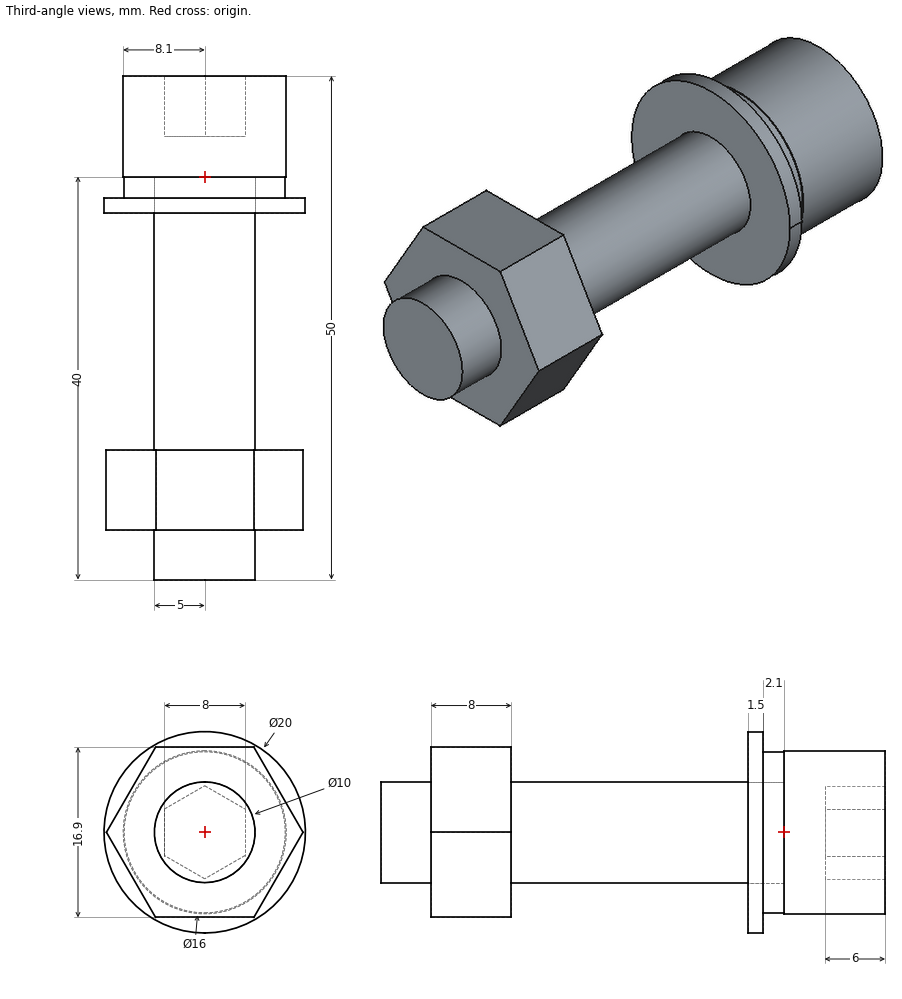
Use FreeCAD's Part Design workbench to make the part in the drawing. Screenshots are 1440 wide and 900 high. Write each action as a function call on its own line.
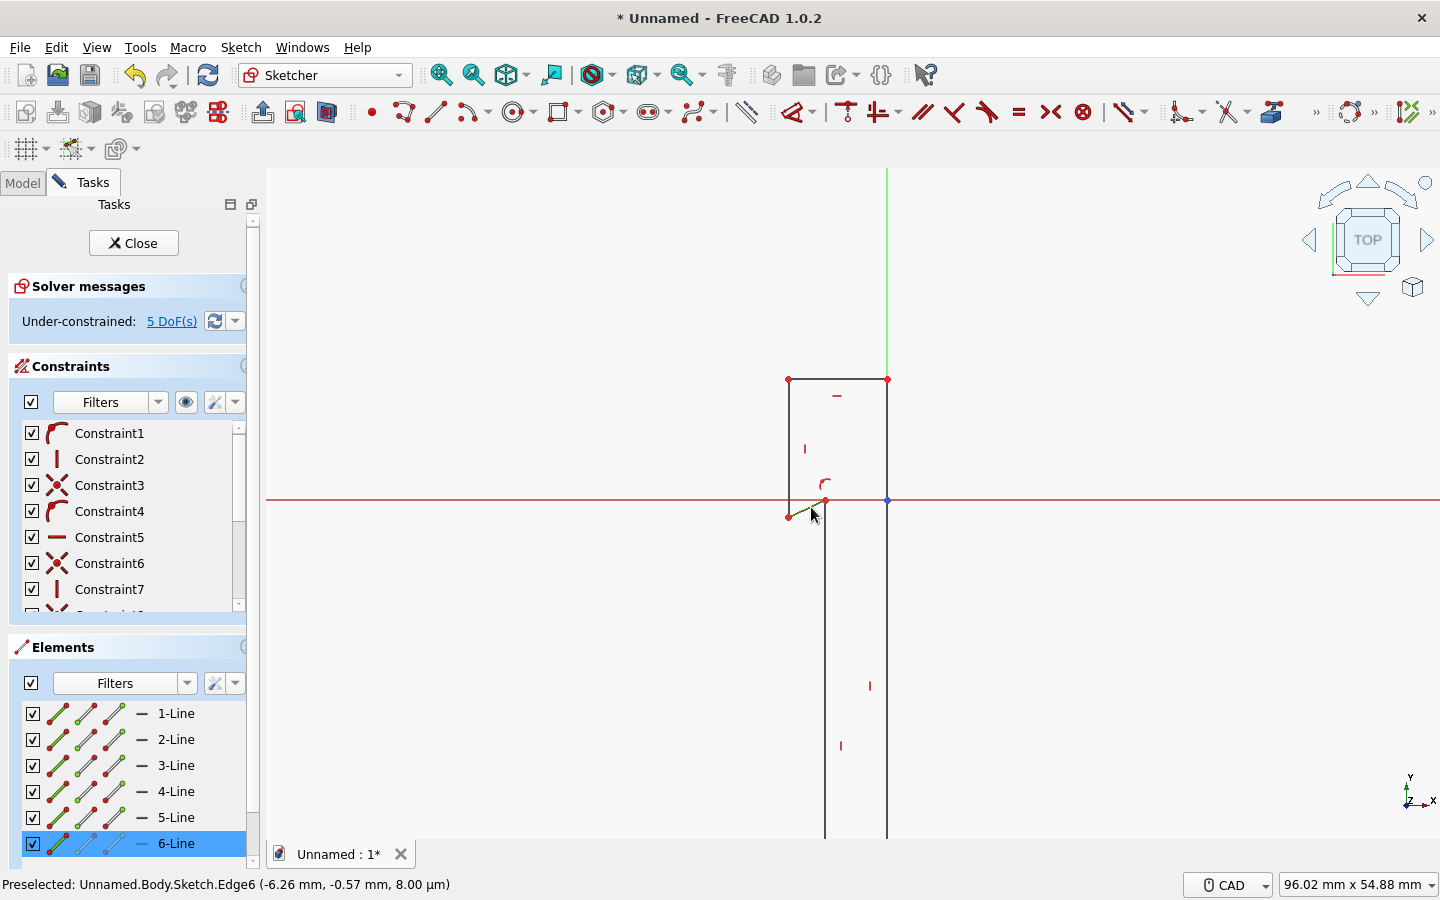
click(900, 112)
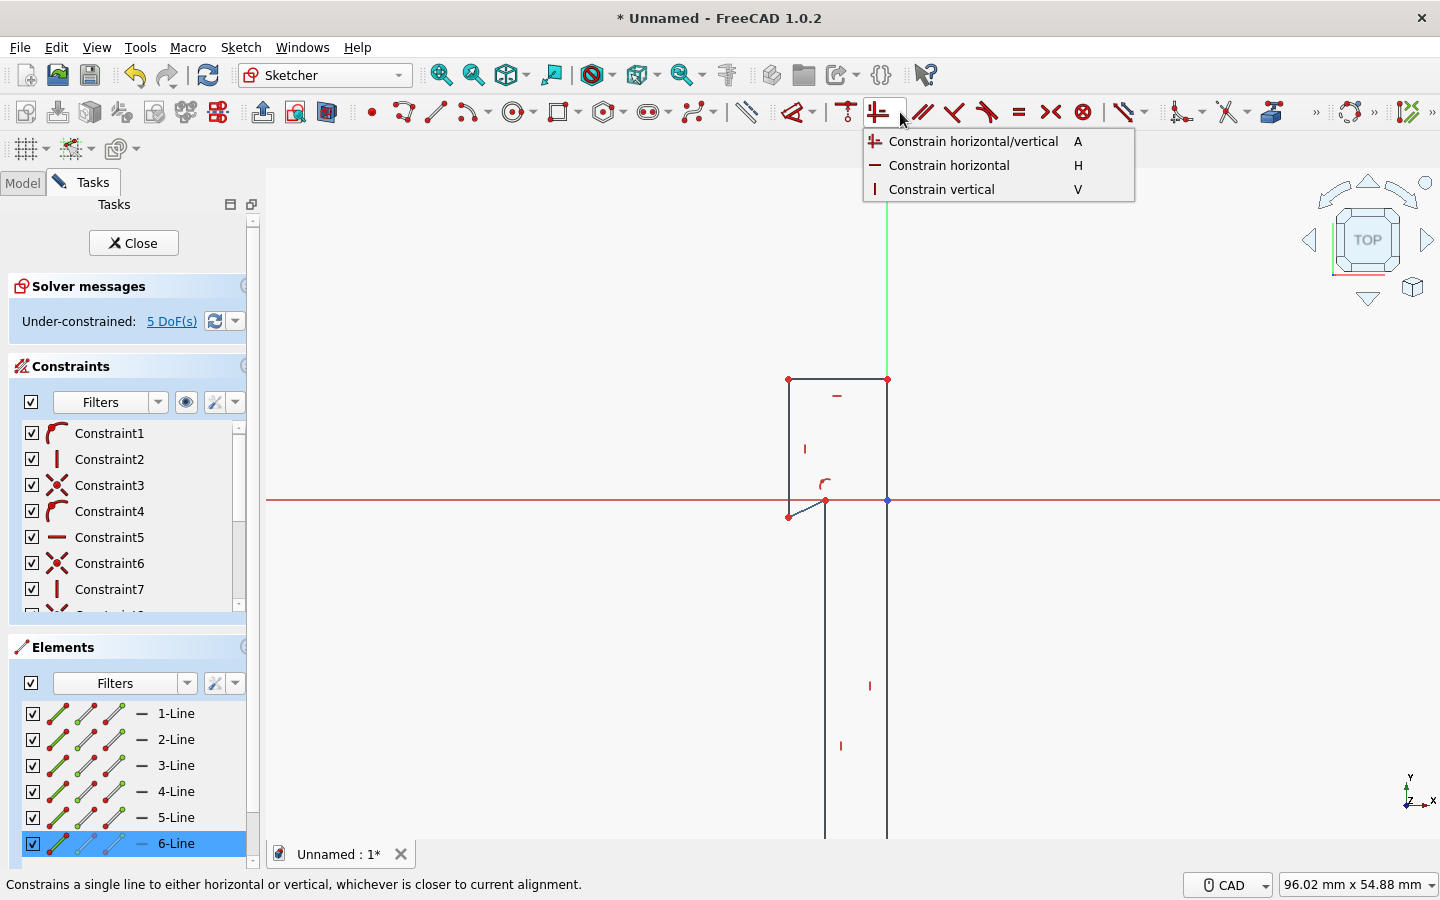
click(999, 165)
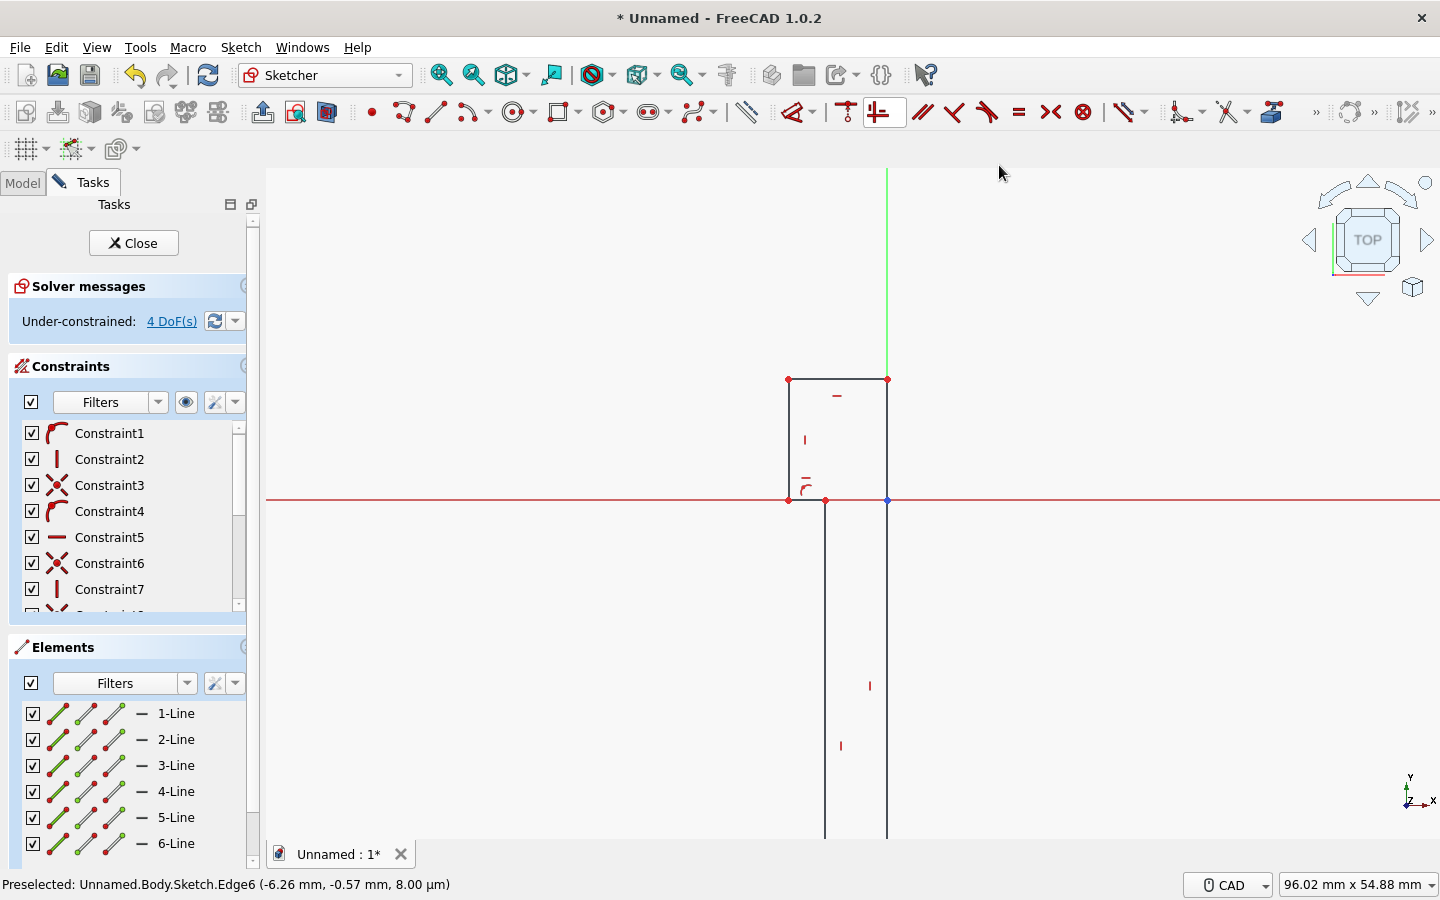
click(792, 112)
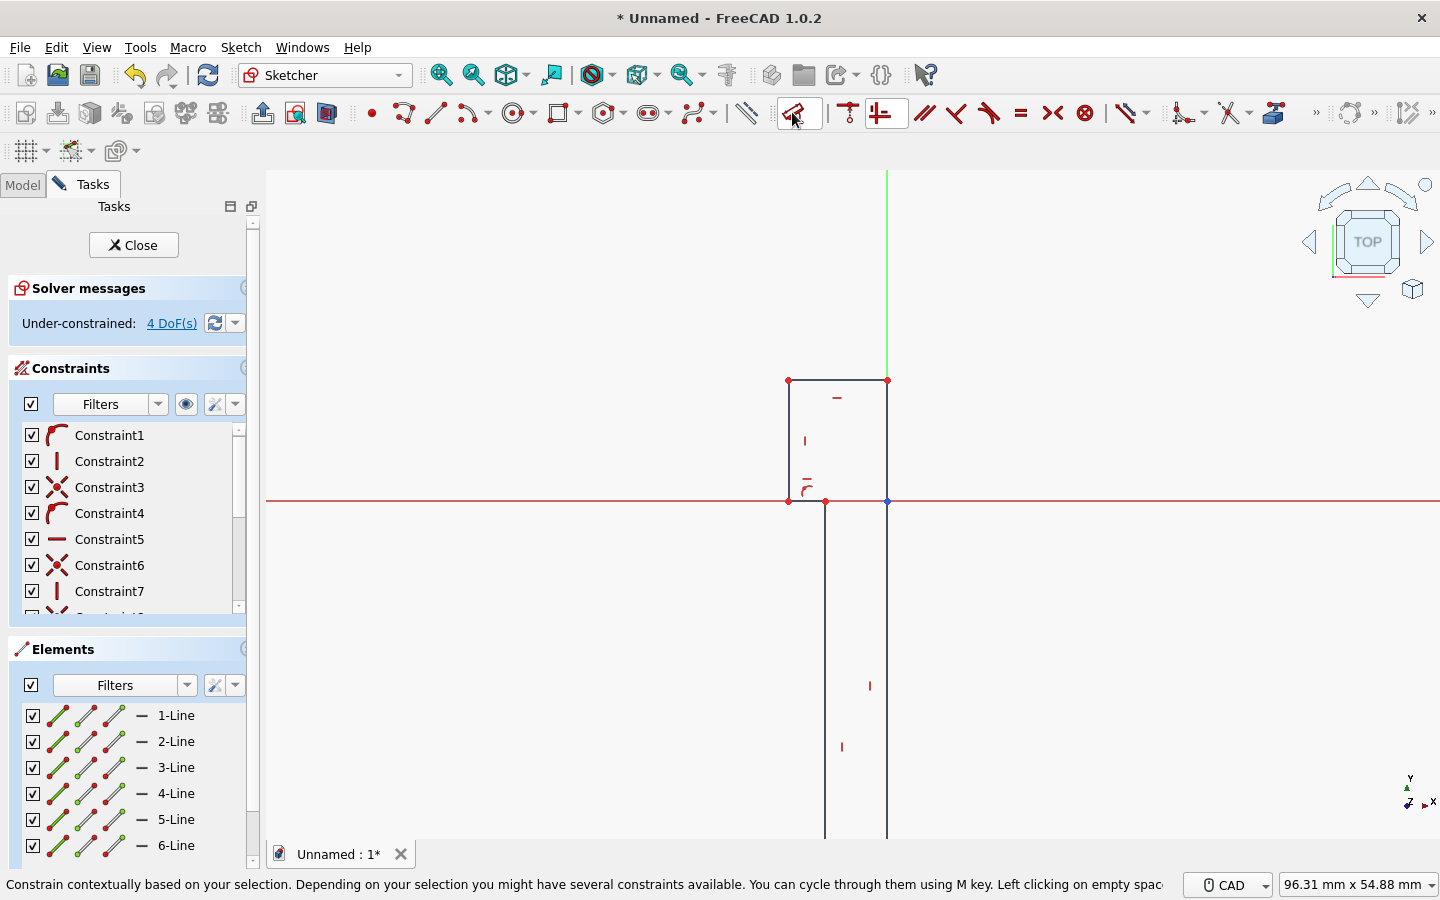
scroll(676, 198, down, 2)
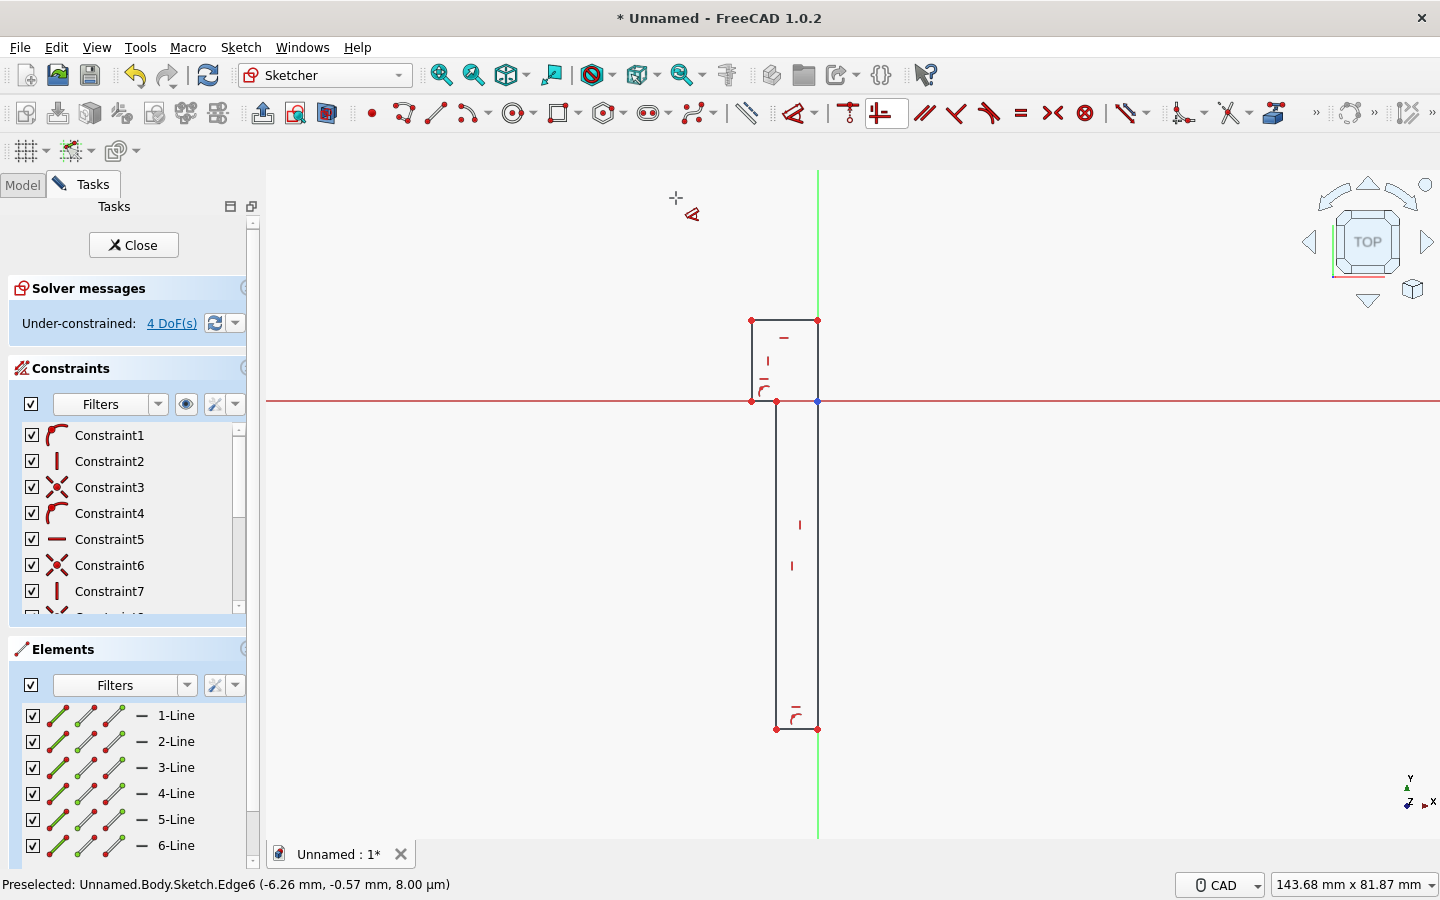
click(789, 729)
click(797, 763)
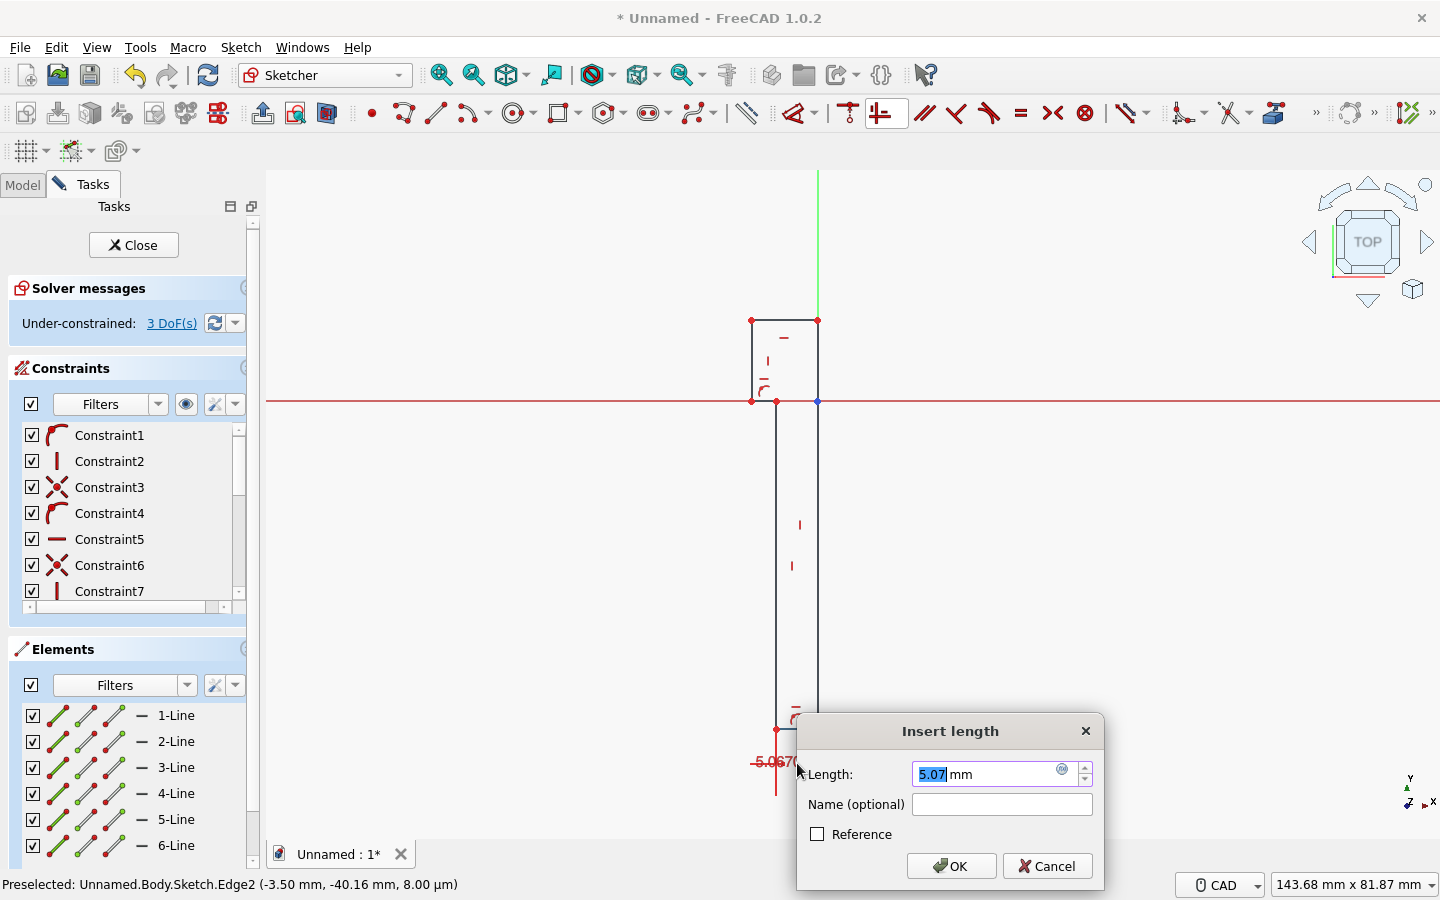
text(5)
key(Return)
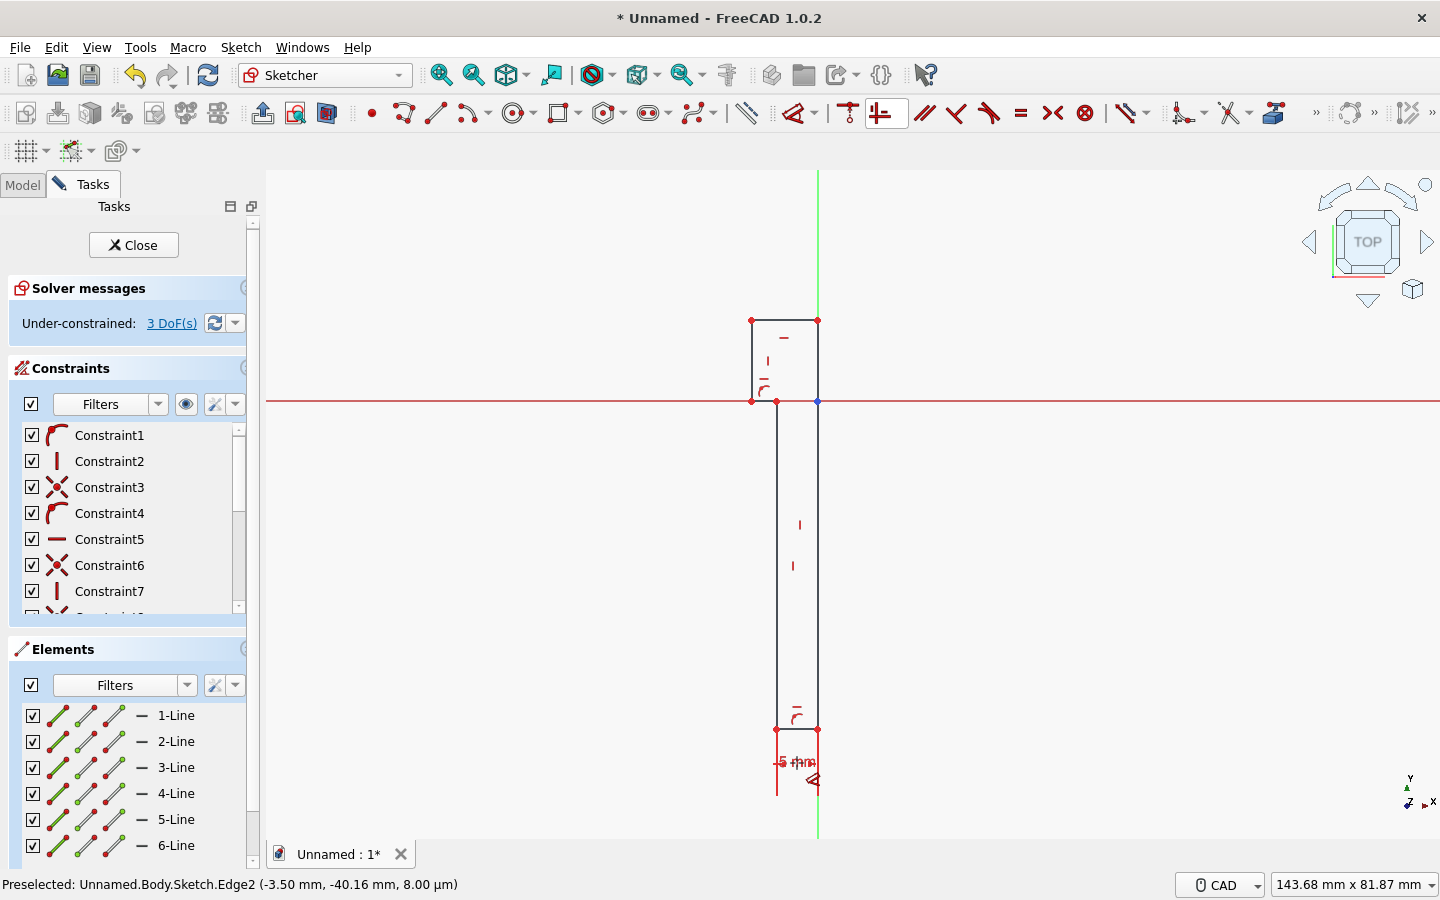
click(777, 500)
click(743, 565)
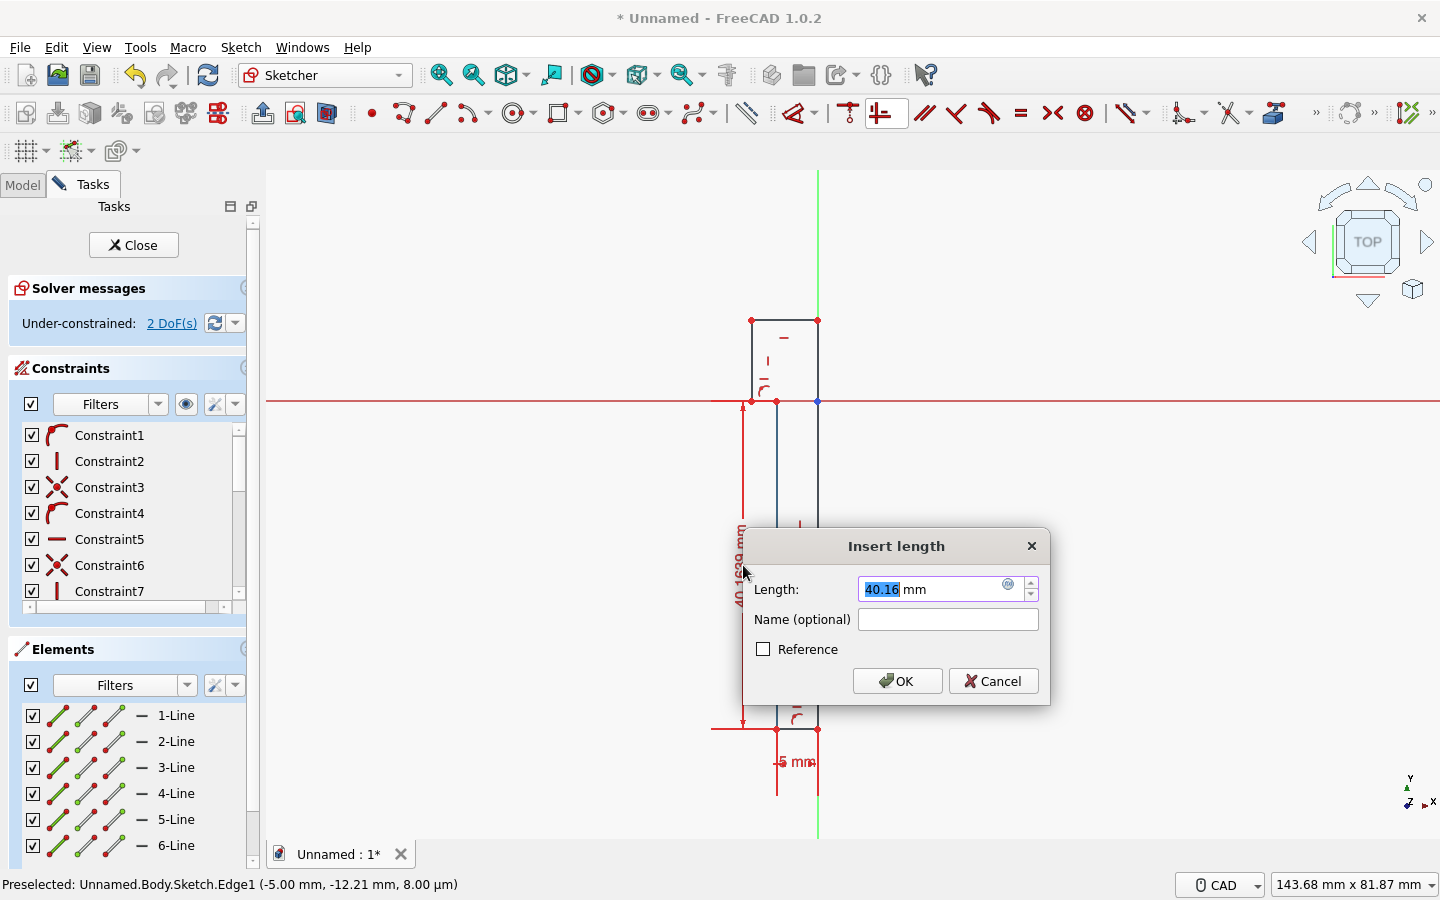
text(40)
key(Return)